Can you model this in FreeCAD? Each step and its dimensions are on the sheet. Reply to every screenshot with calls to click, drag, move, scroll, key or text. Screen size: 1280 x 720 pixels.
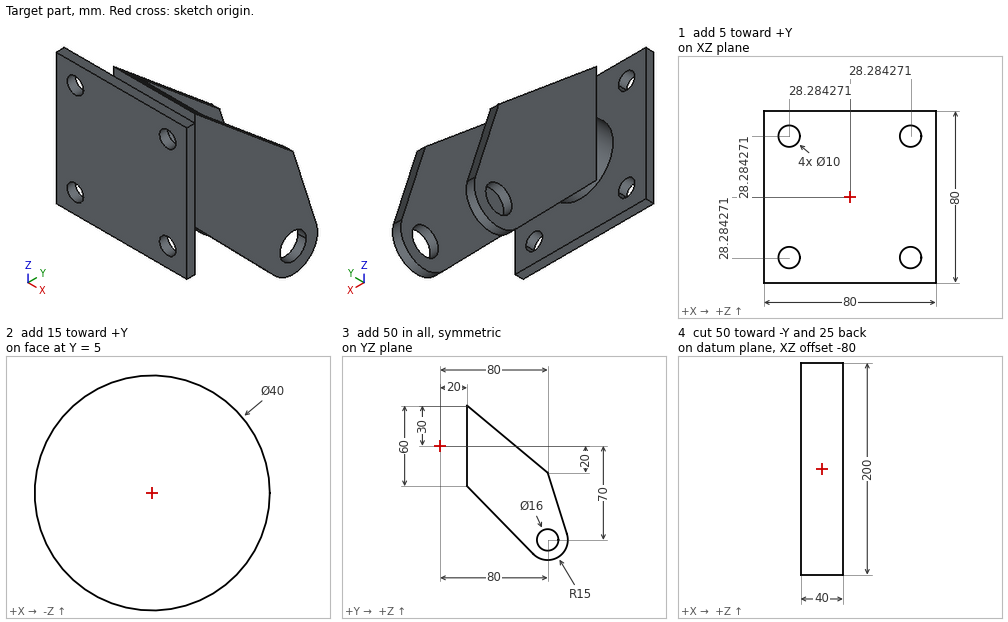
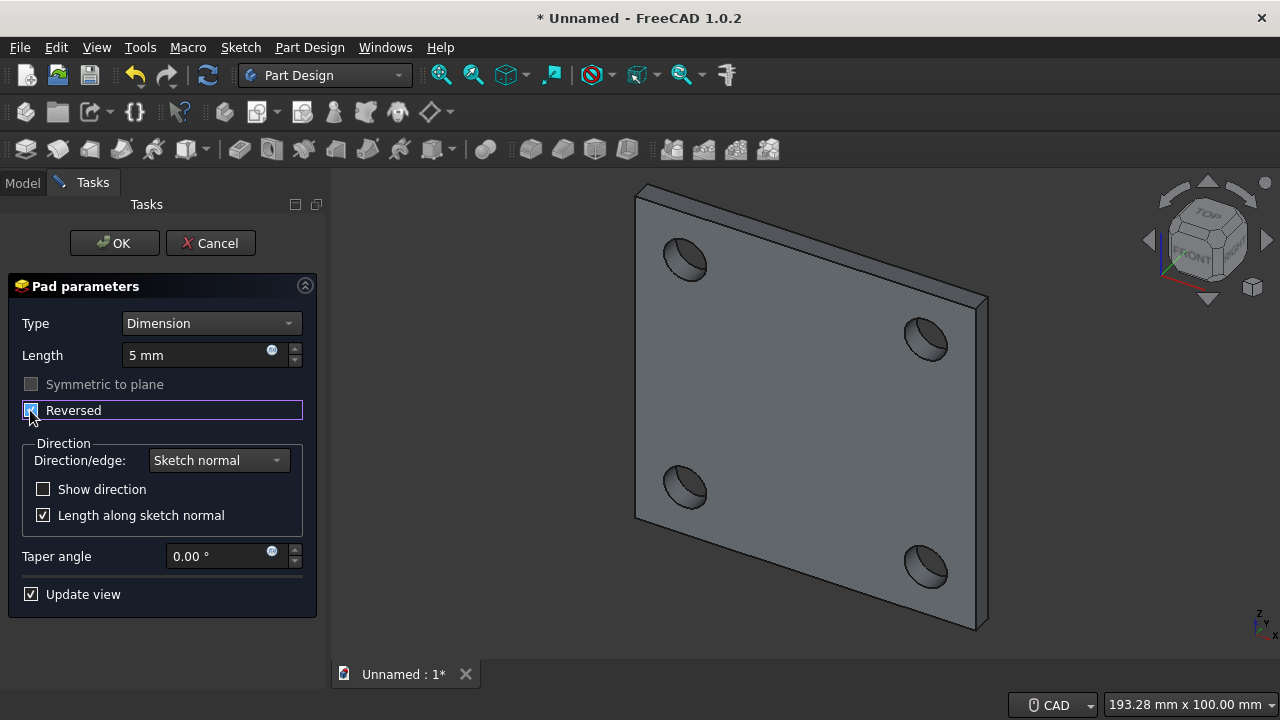
click(115, 243)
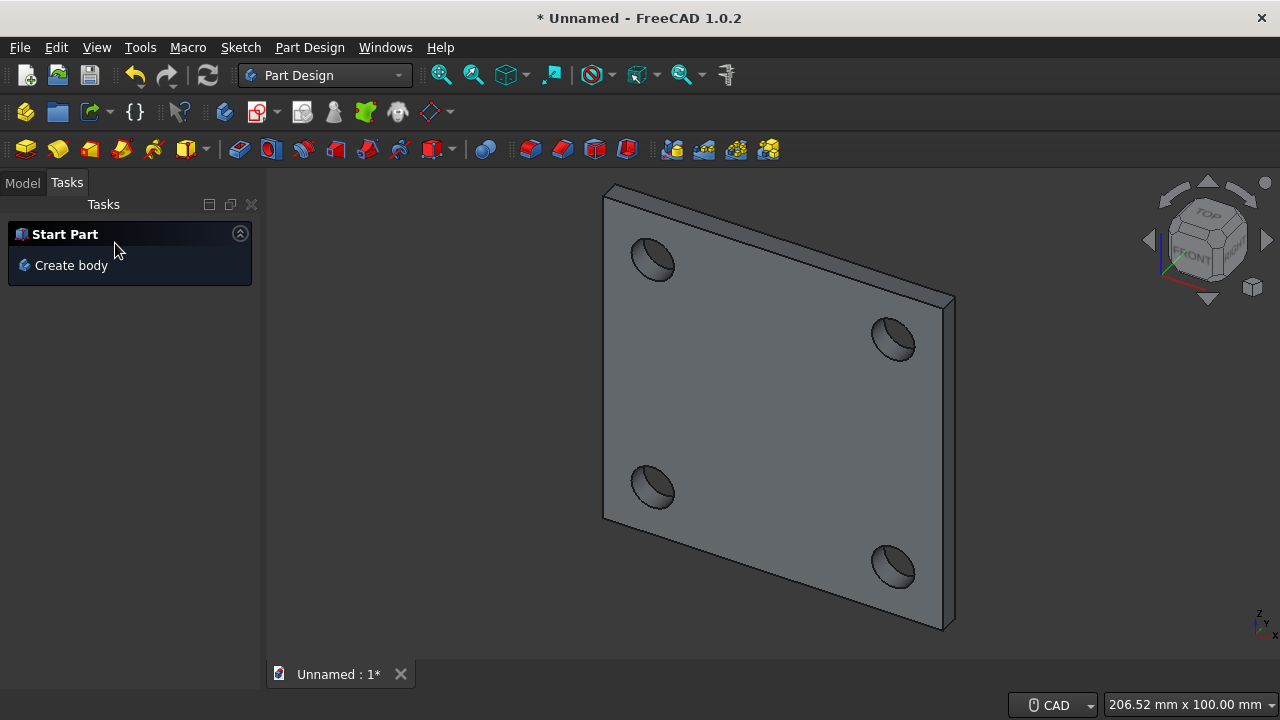
key(4)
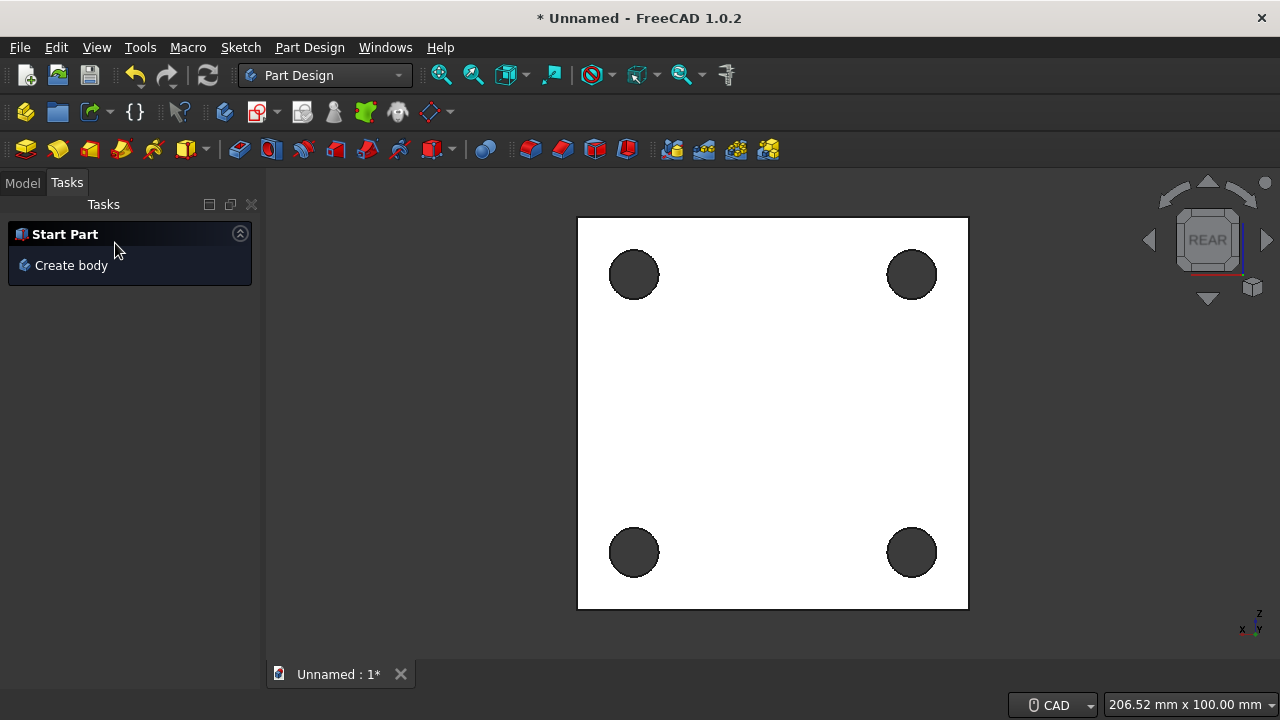
click(773, 412)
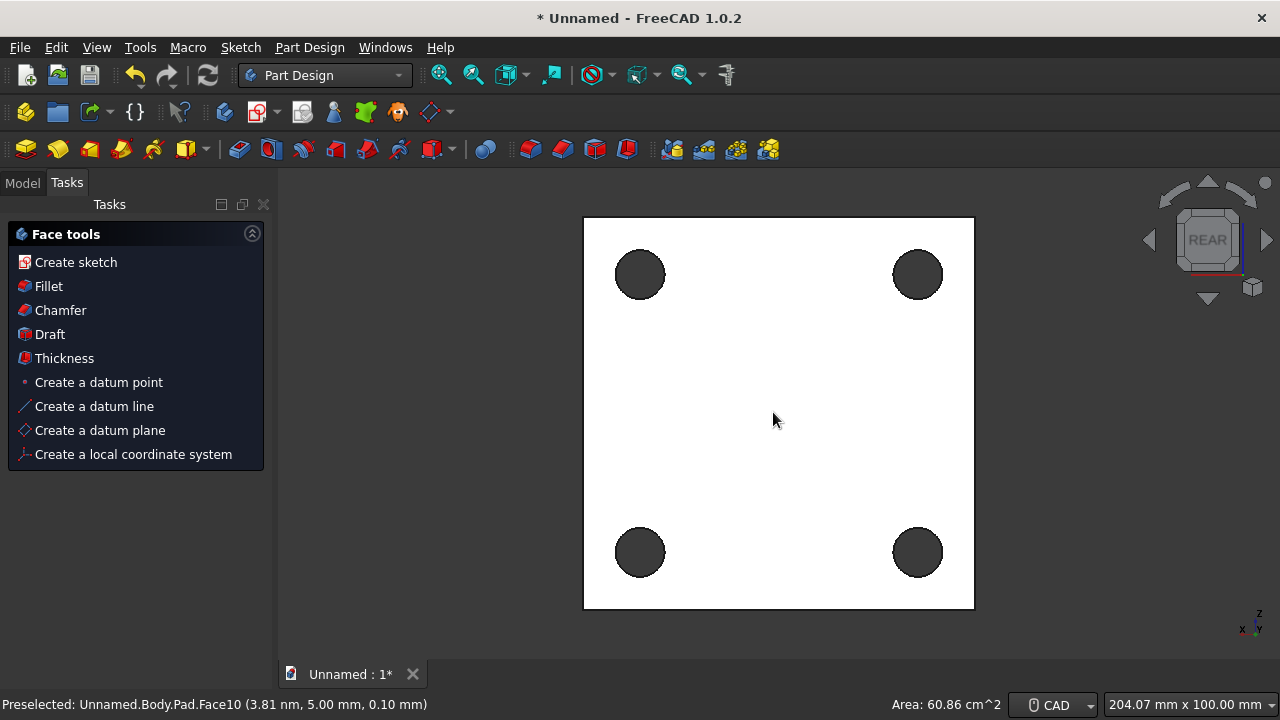
click(258, 112)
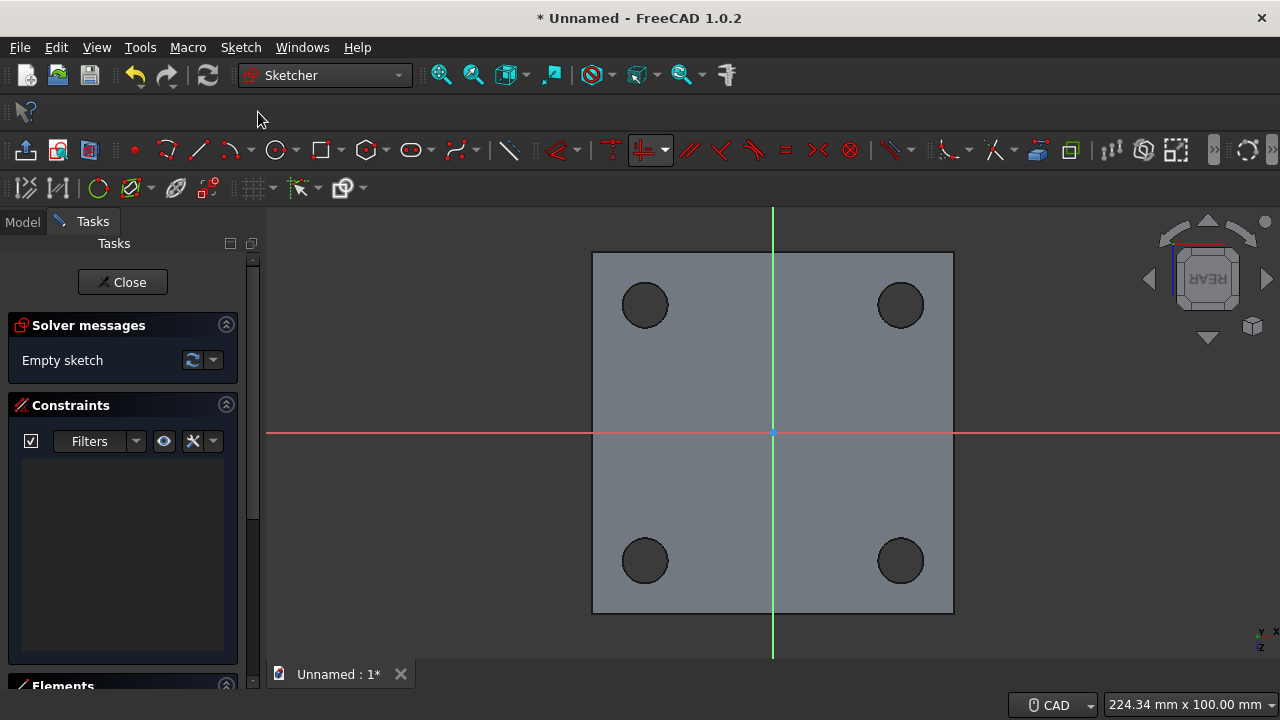
scroll(912, 433, up, 2)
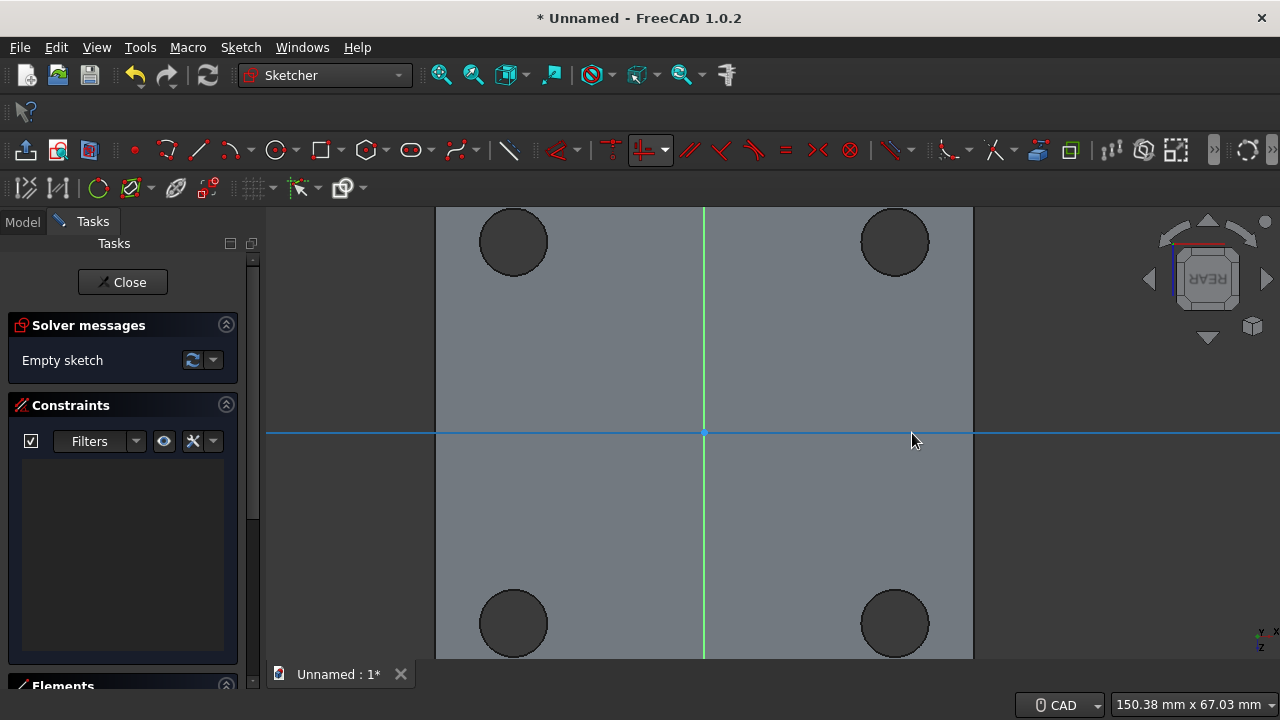
click(276, 150)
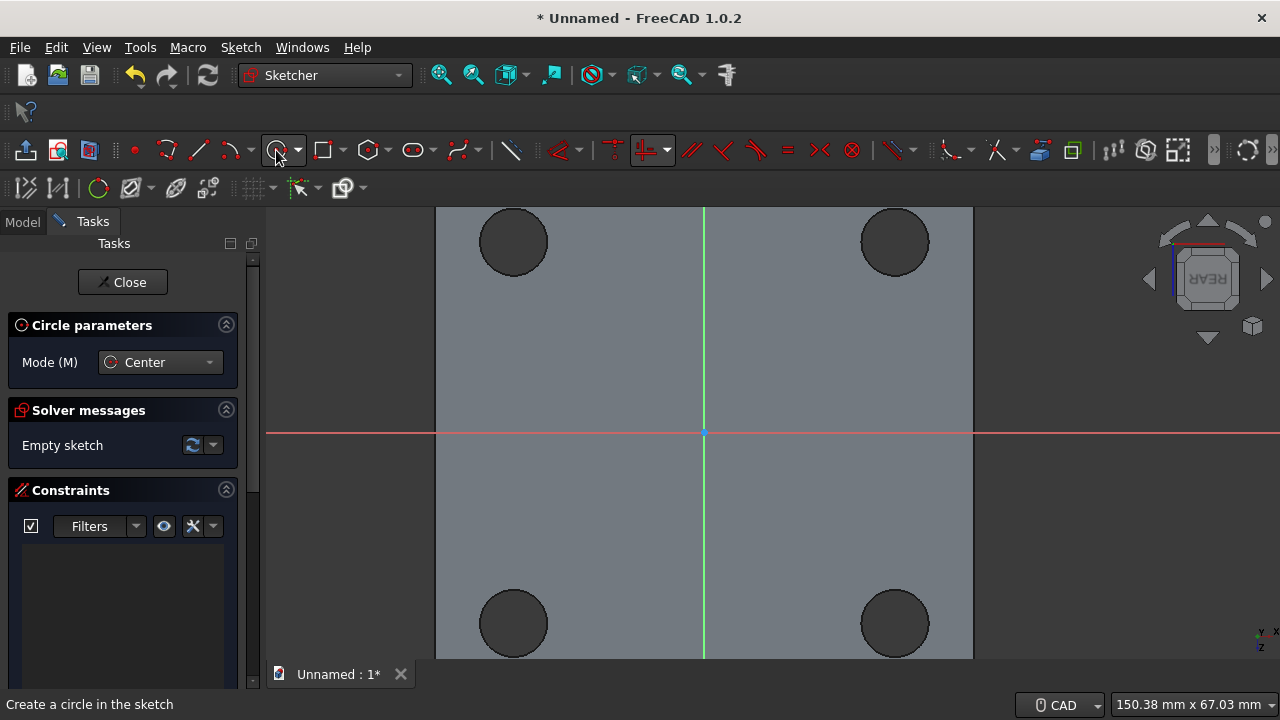
click(704, 433)
click(800, 337)
key(Escape)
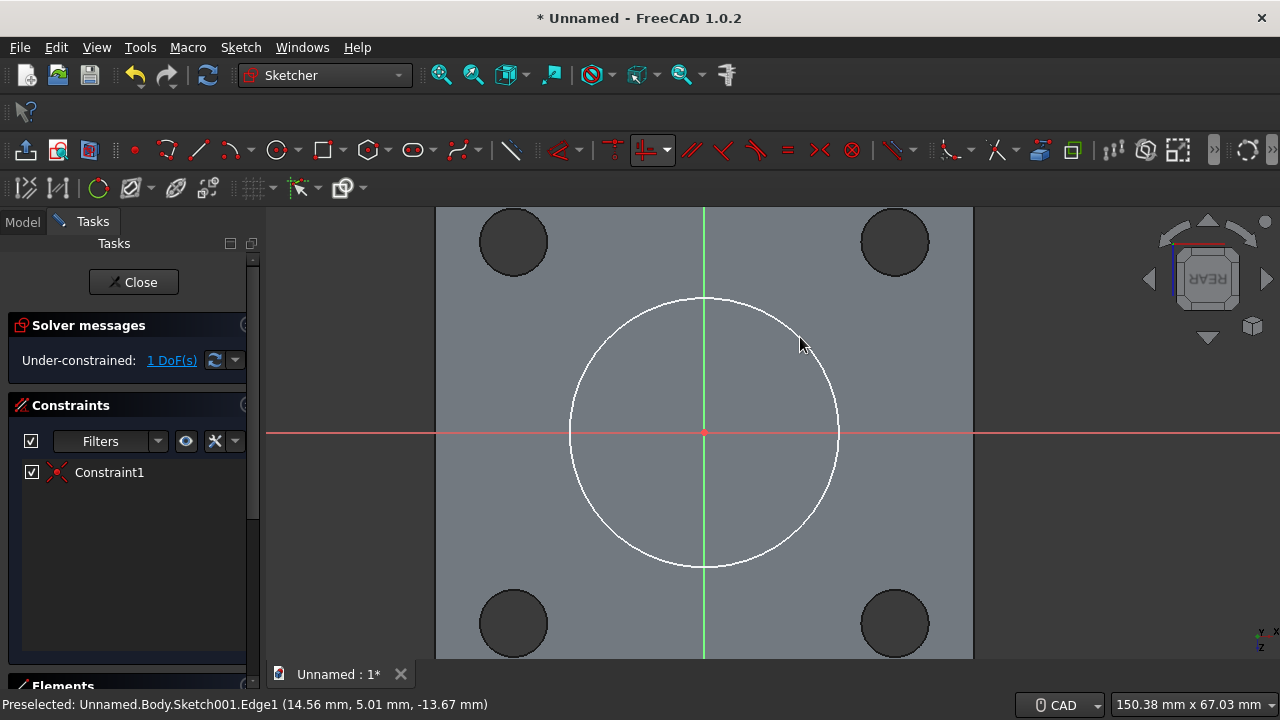
click(558, 150)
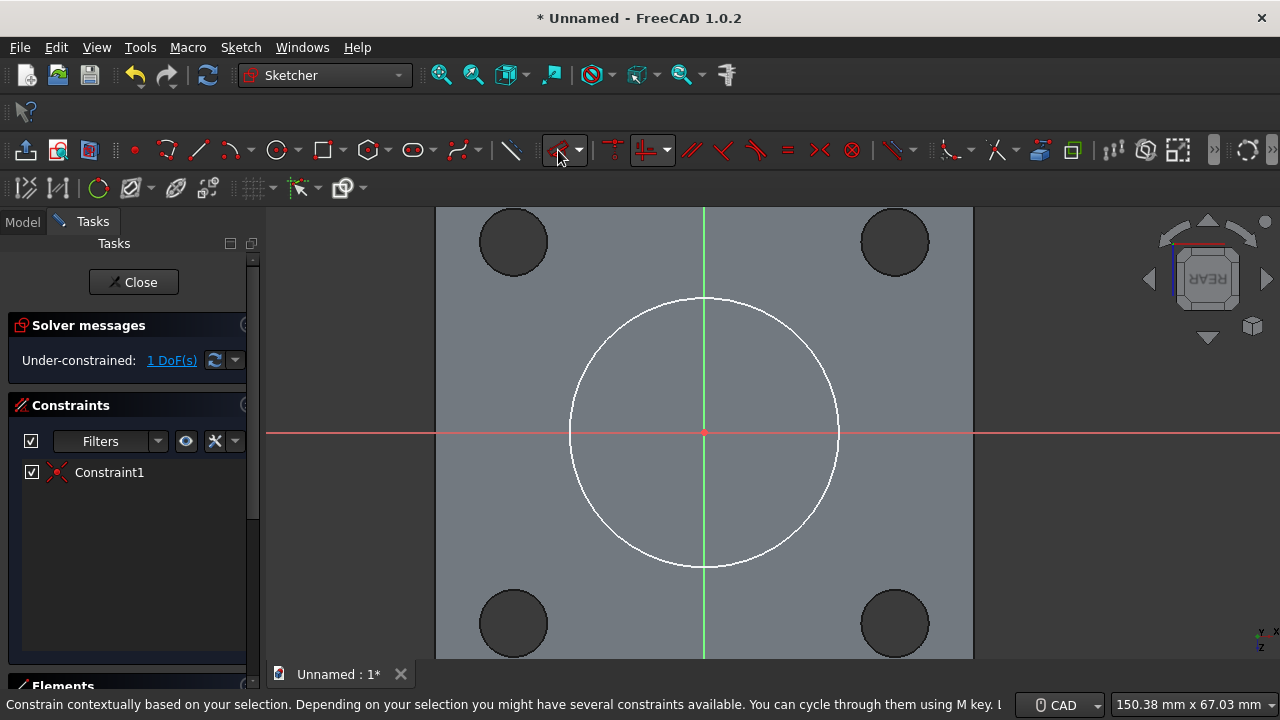
click(799, 337)
click(821, 314)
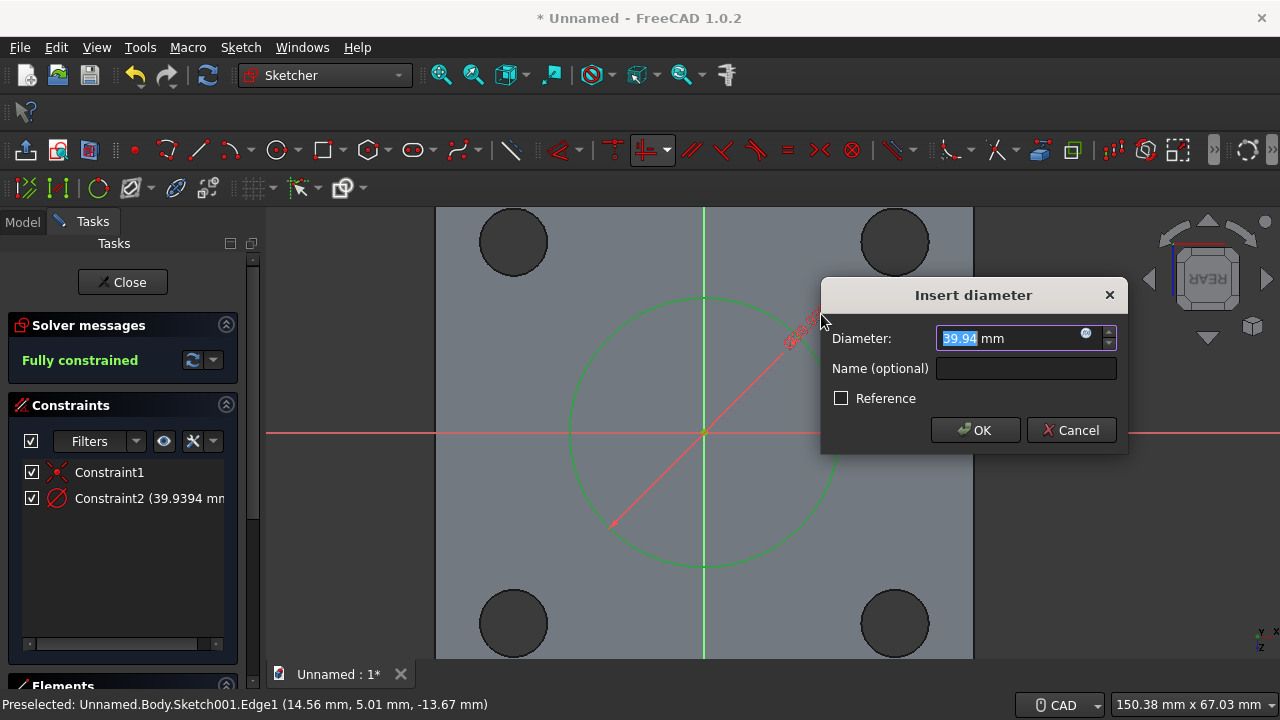
text(40)
key(Return)
key(Escape)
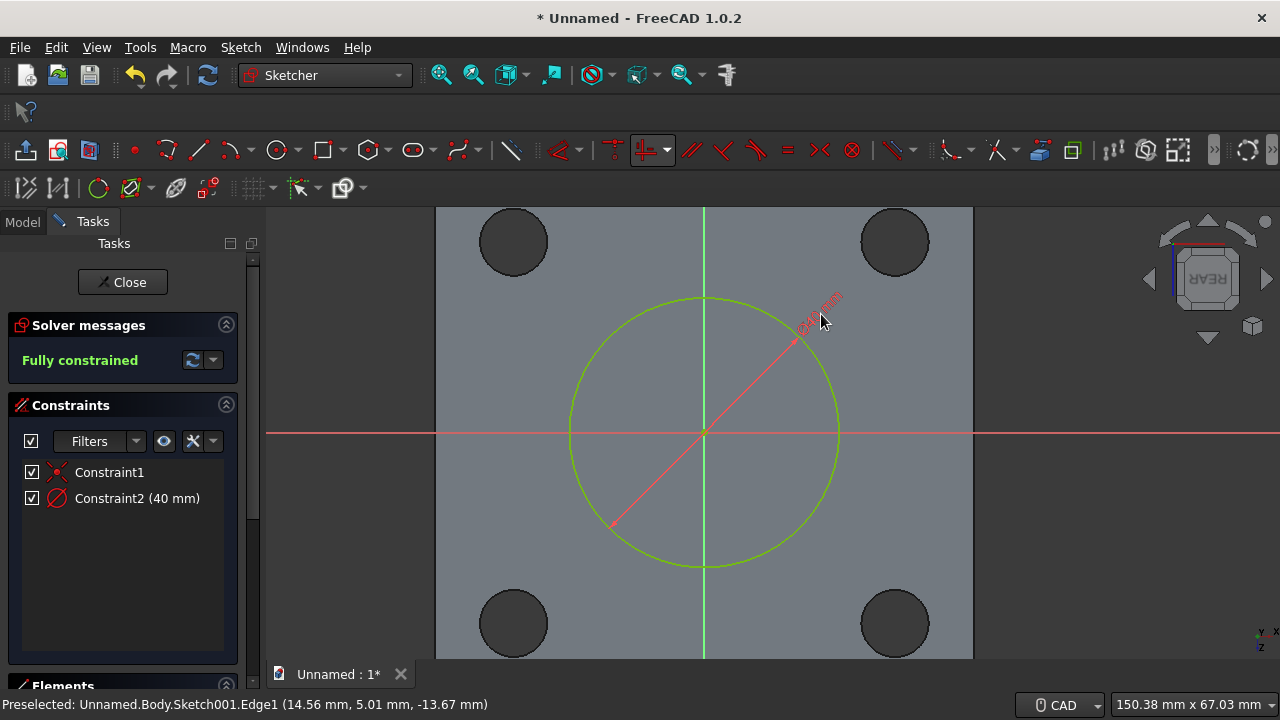
click(123, 282)